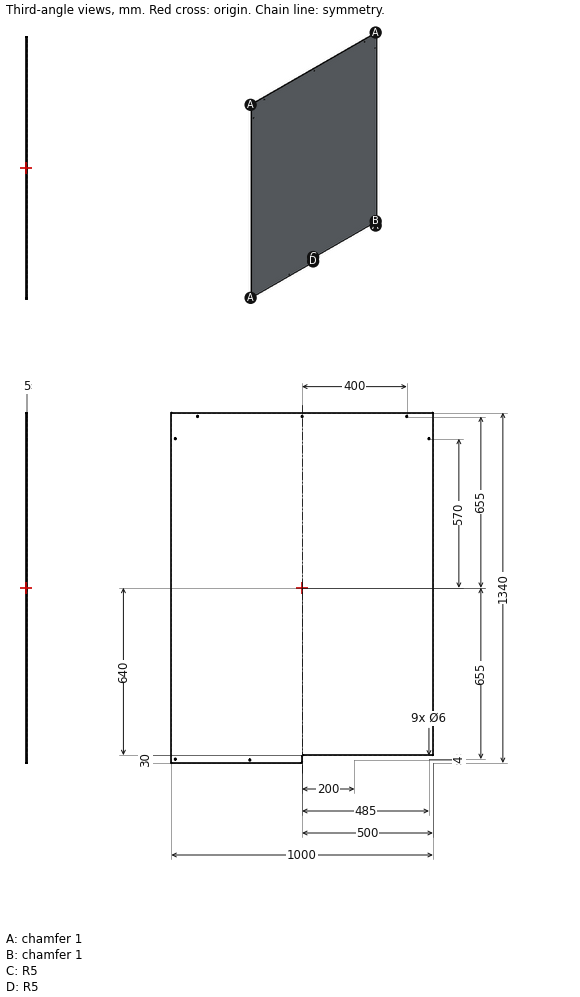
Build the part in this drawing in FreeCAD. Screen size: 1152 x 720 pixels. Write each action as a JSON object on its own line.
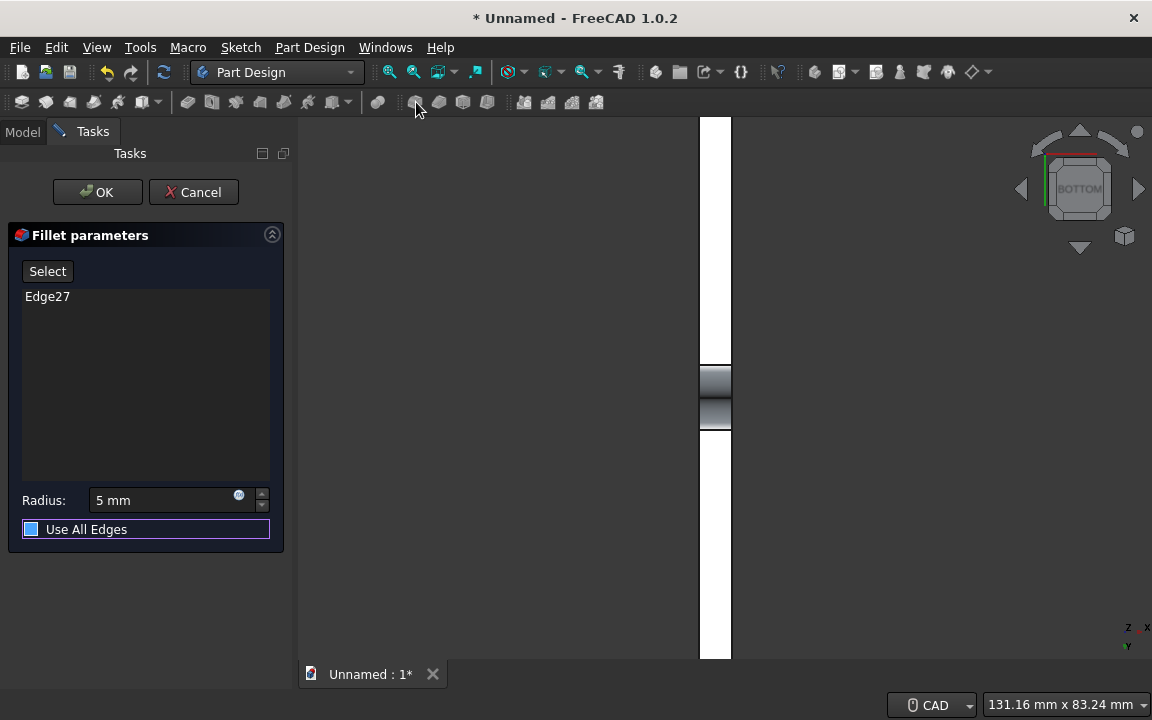
{"action": "left_click", "coordinate": [98, 192]}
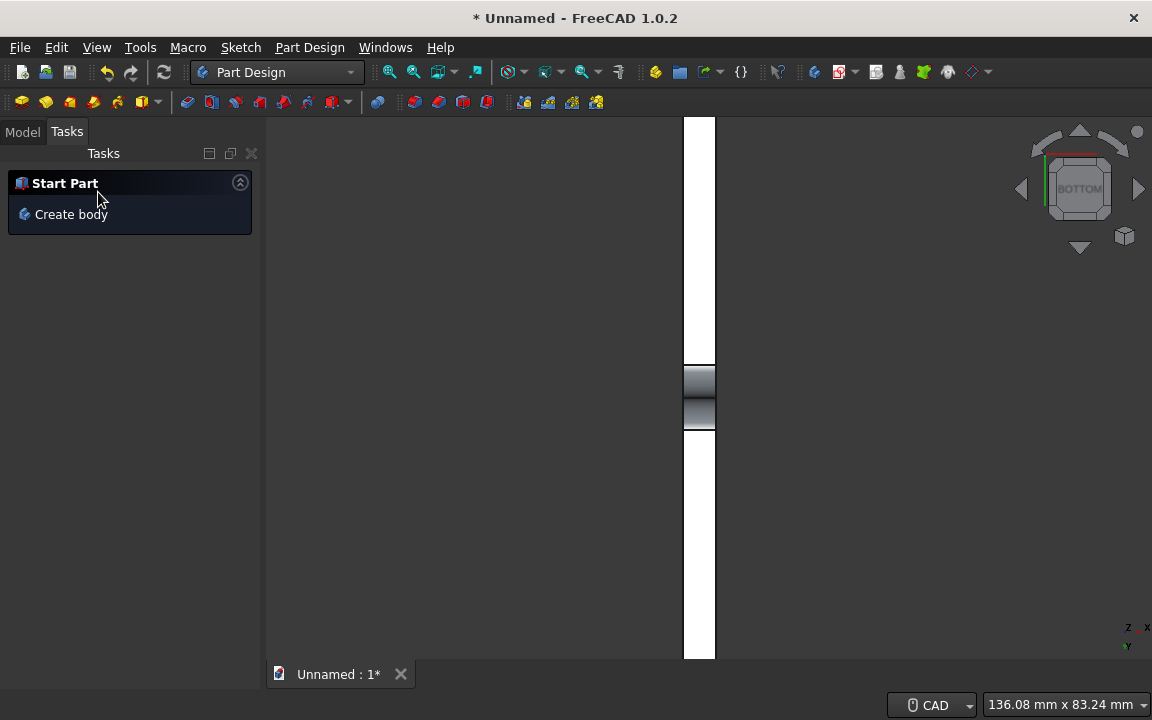
{"action": "key", "text": "0"}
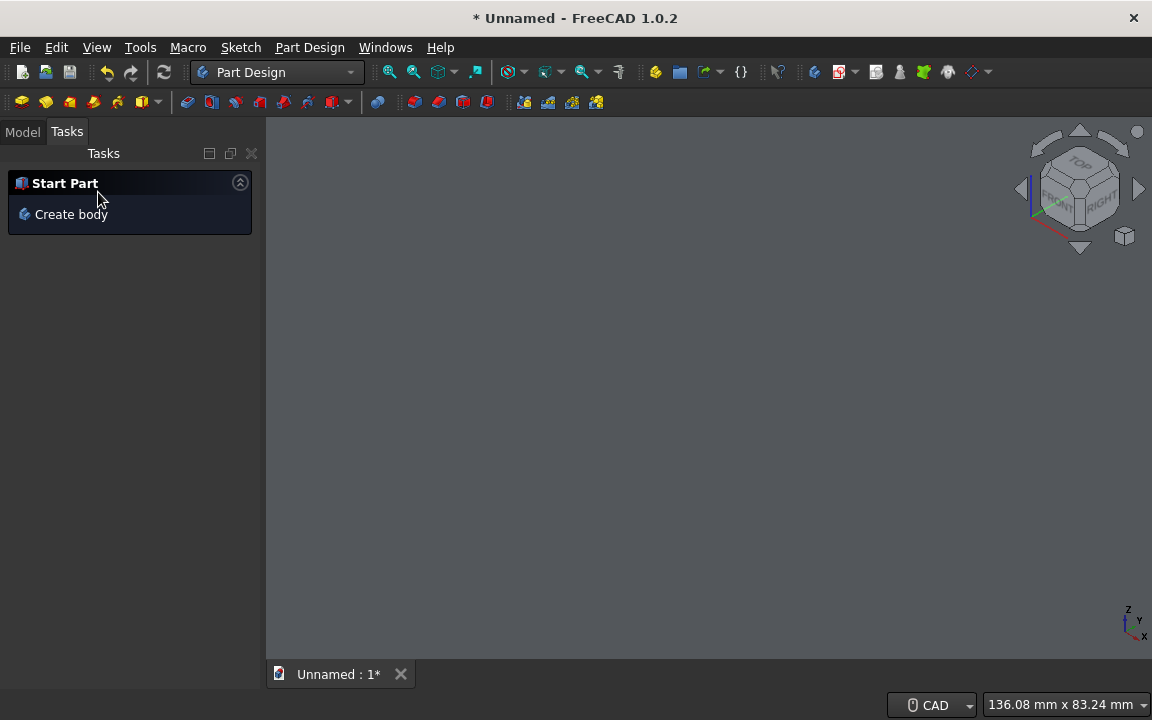
{"action": "left_click", "coordinate": [390, 72]}